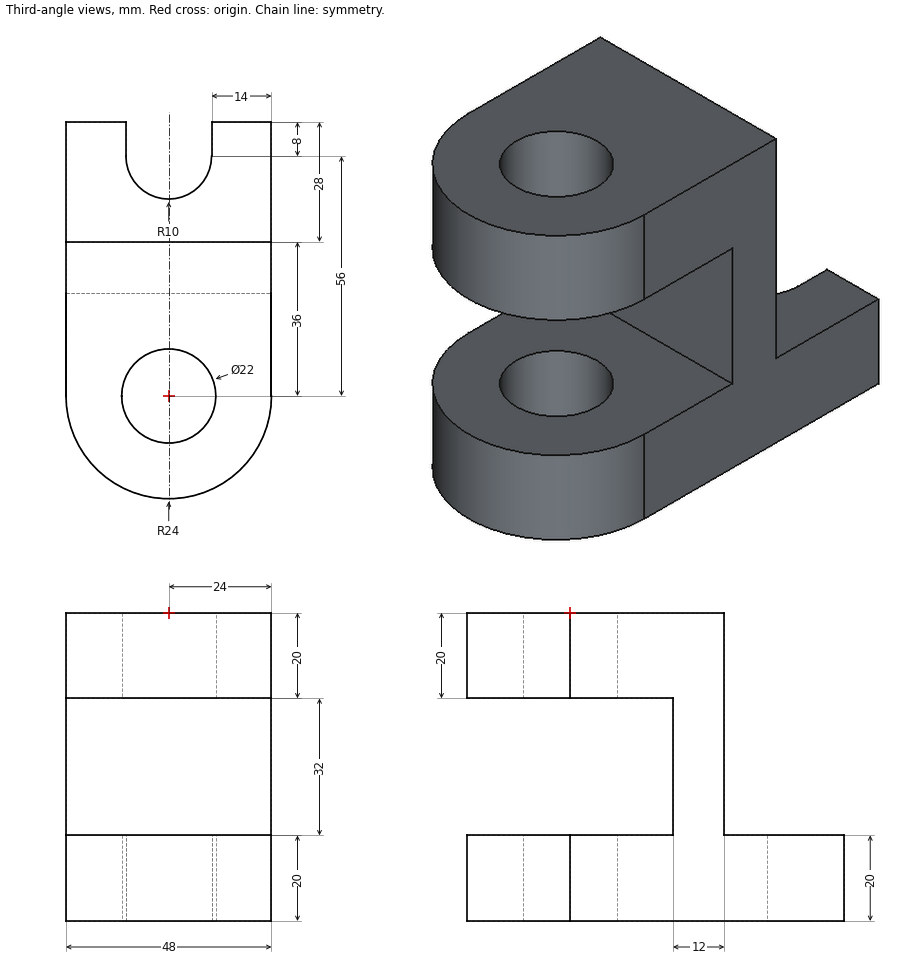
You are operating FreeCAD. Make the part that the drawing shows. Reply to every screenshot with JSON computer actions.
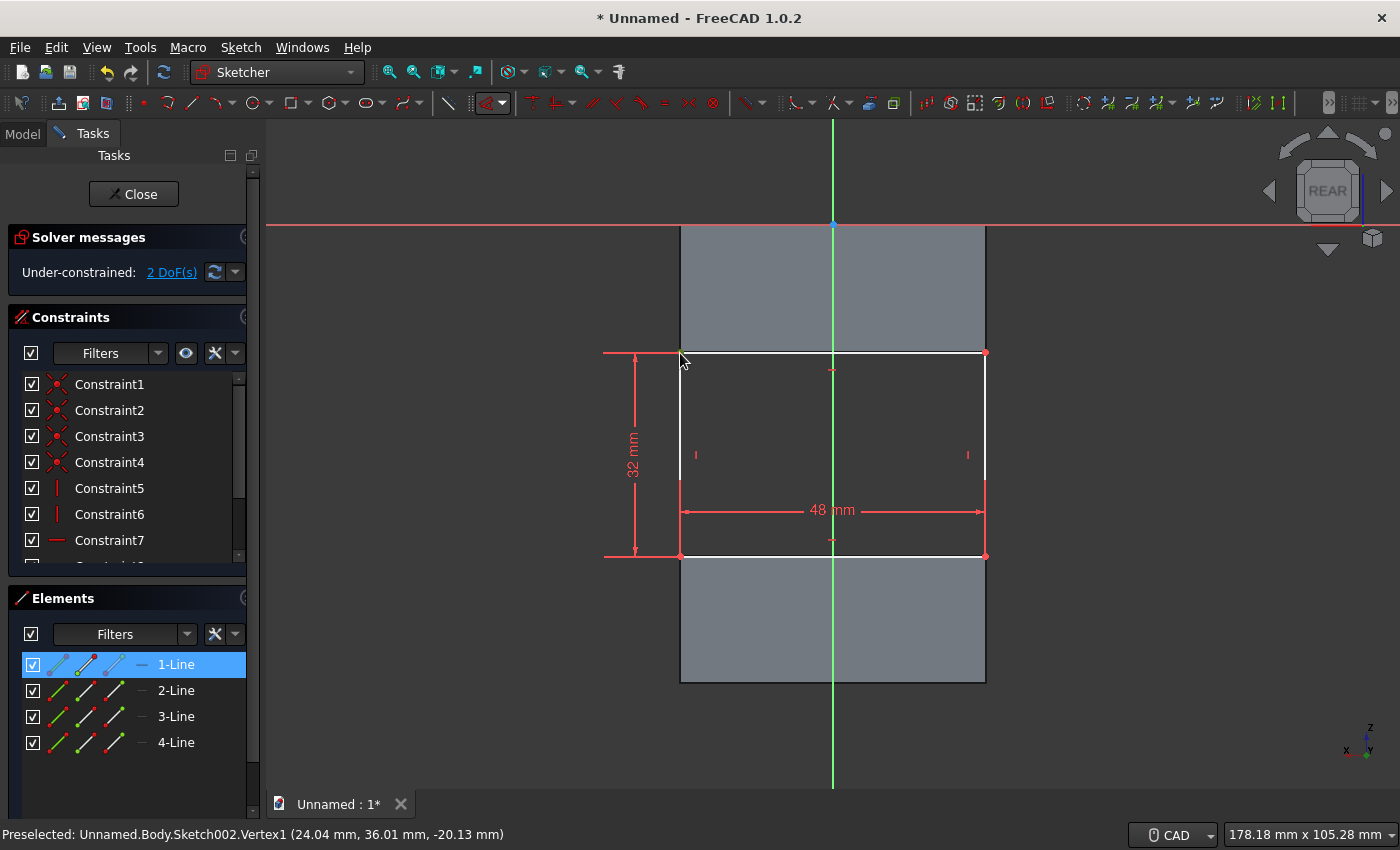
{"action": "left_click", "coordinate": [504, 104]}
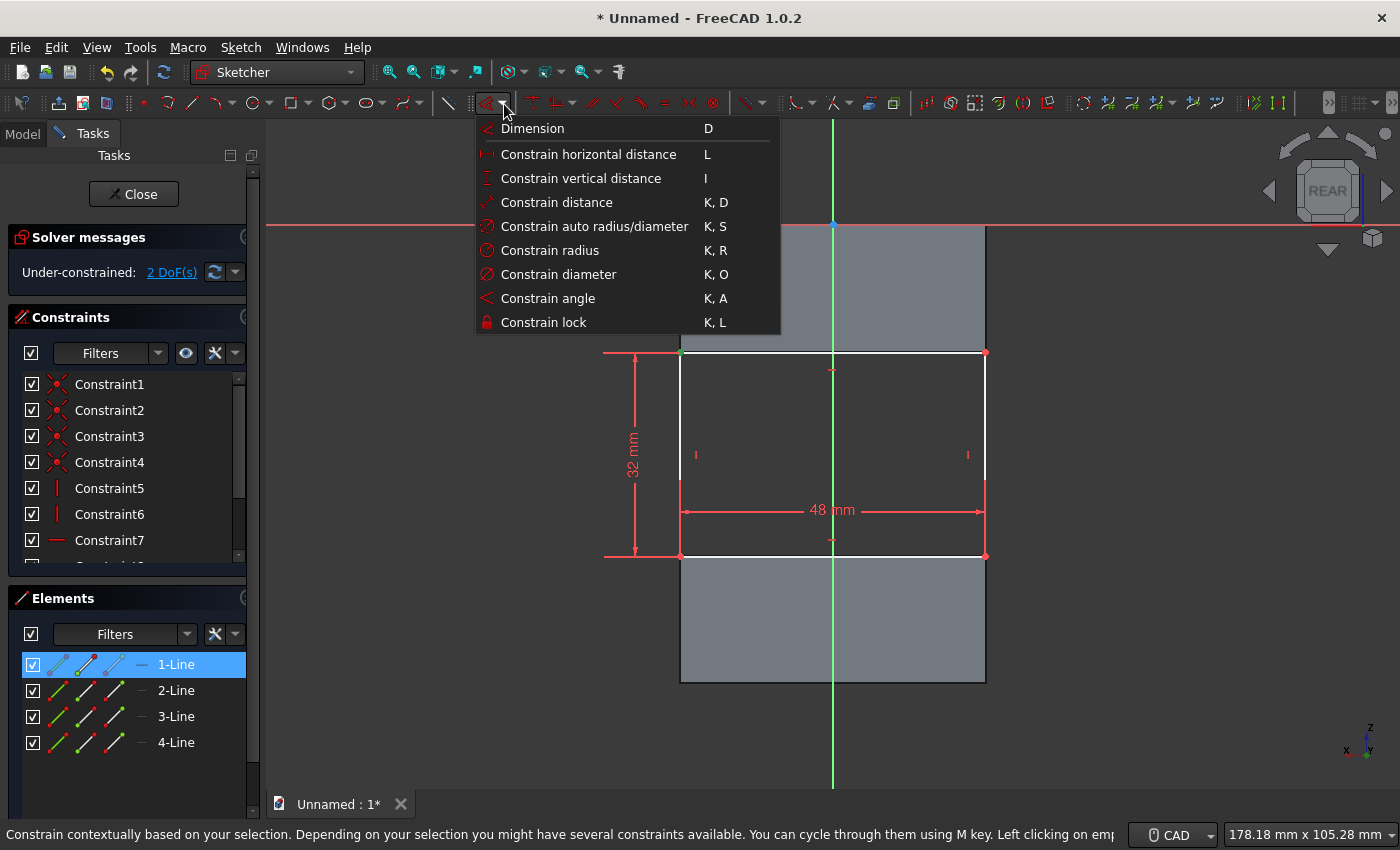
{"action": "left_click", "coordinate": [628, 154]}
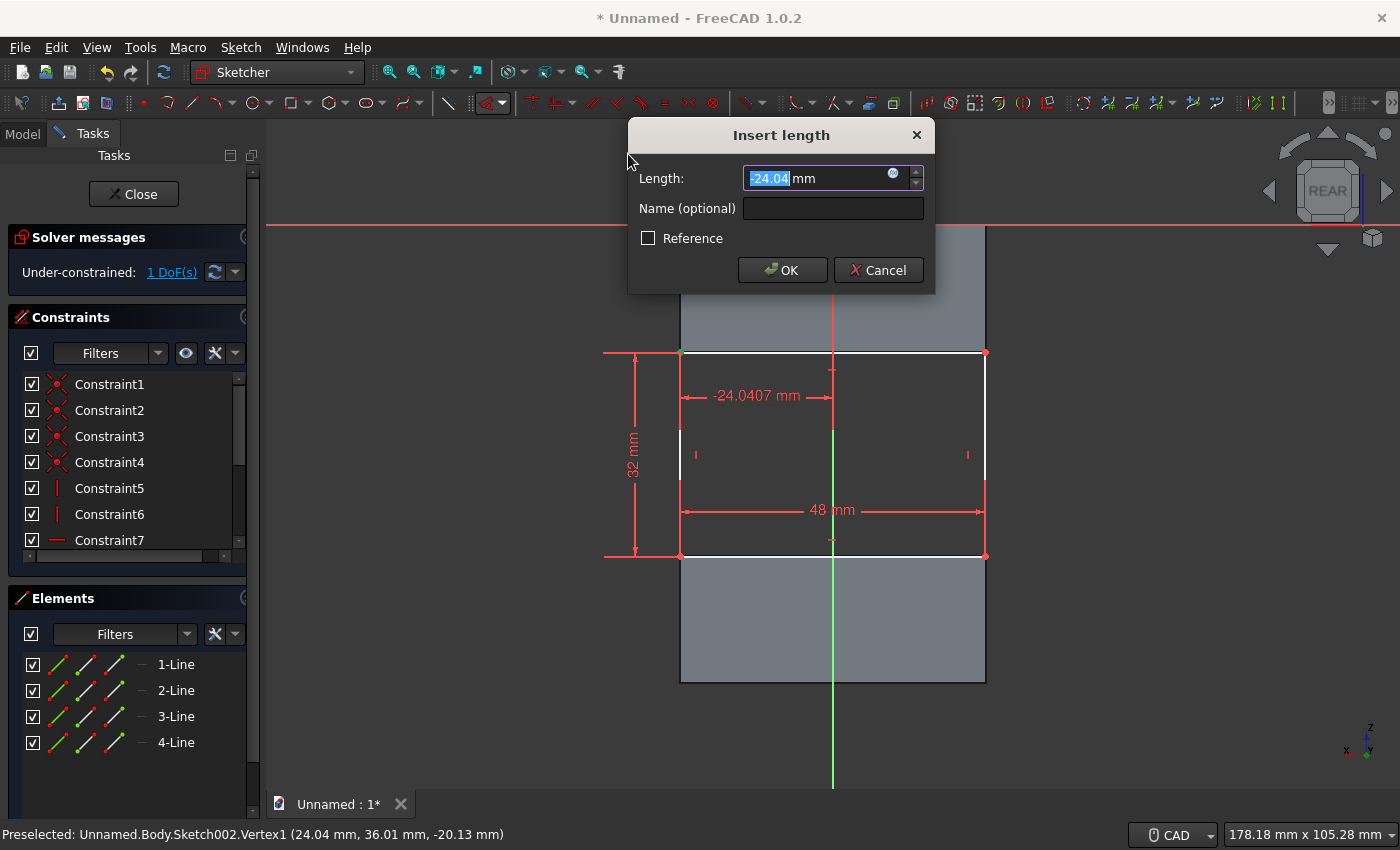
{"action": "type", "text": "-24"}
{"action": "key", "text": "Return"}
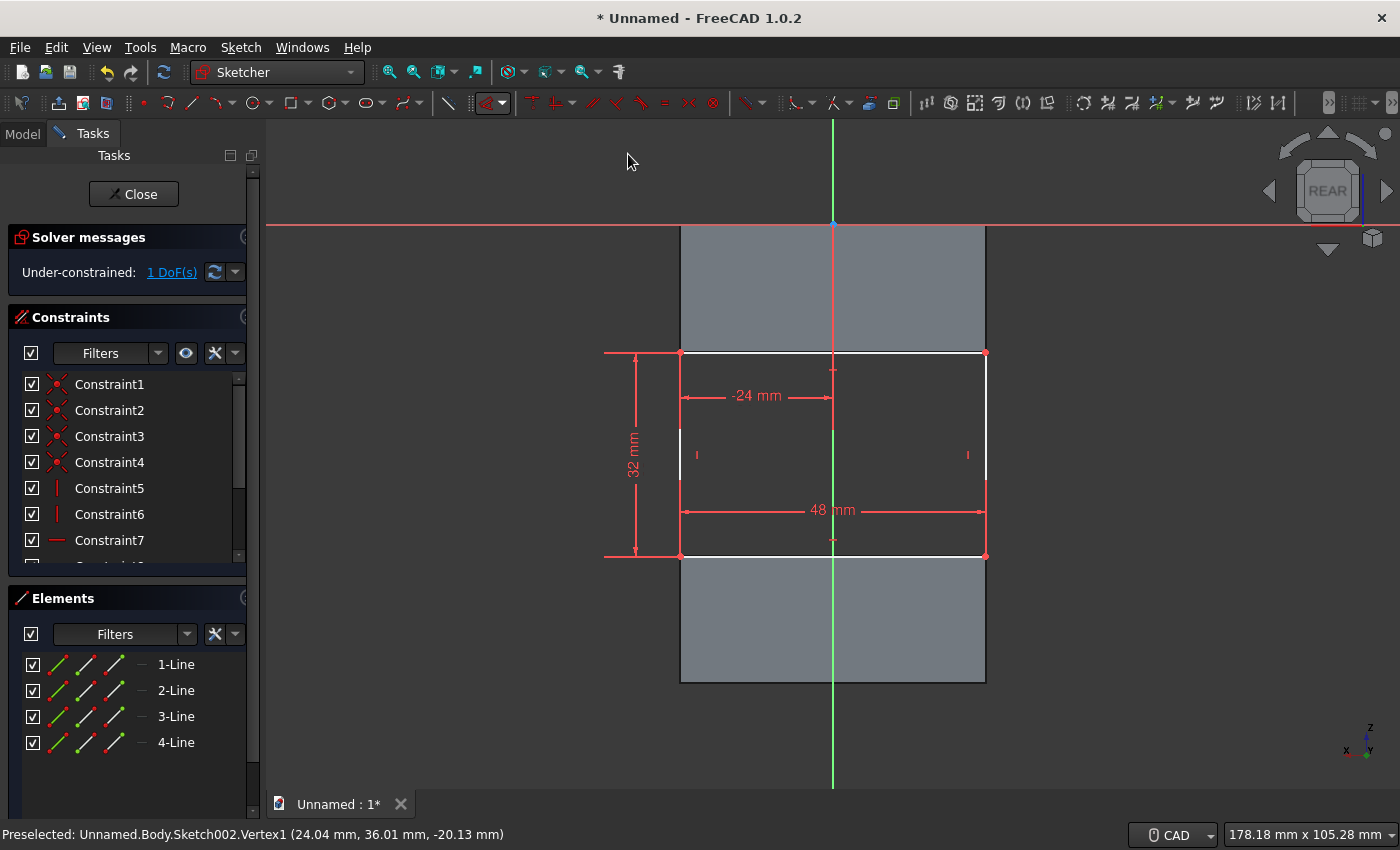
{"action": "left_click", "coordinate": [680, 353]}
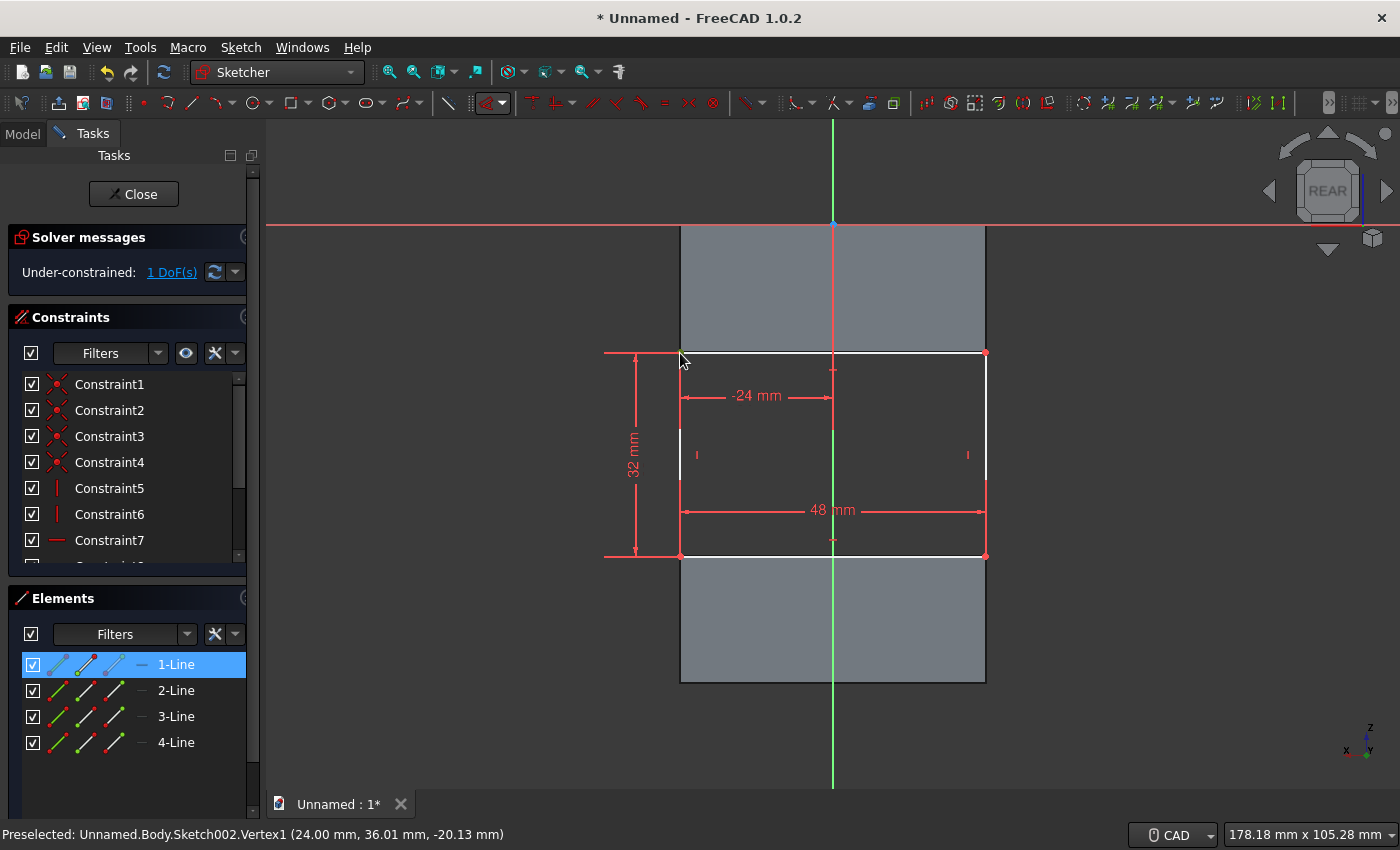
{"action": "left_click", "coordinate": [504, 104]}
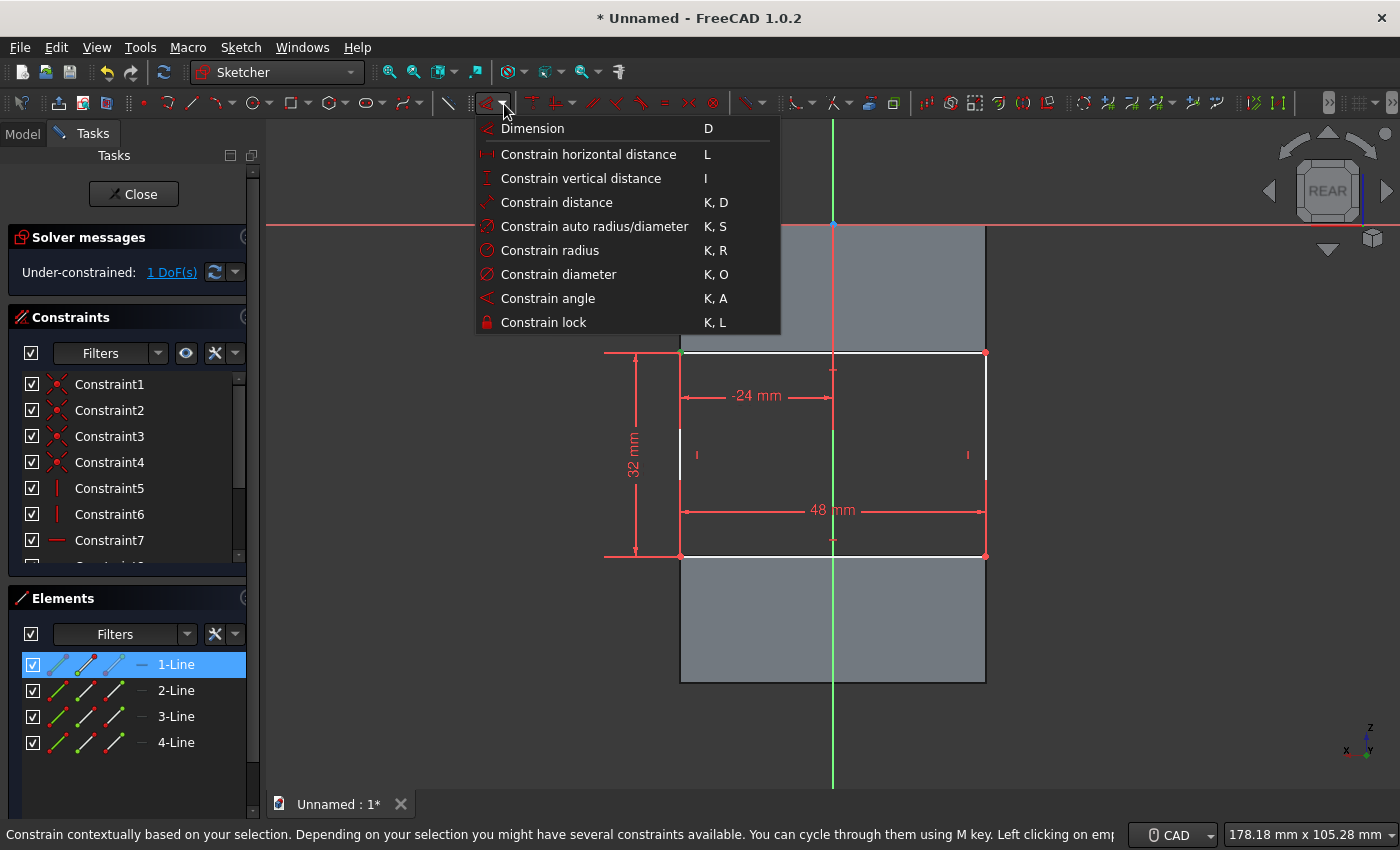
{"action": "left_click", "coordinate": [628, 178]}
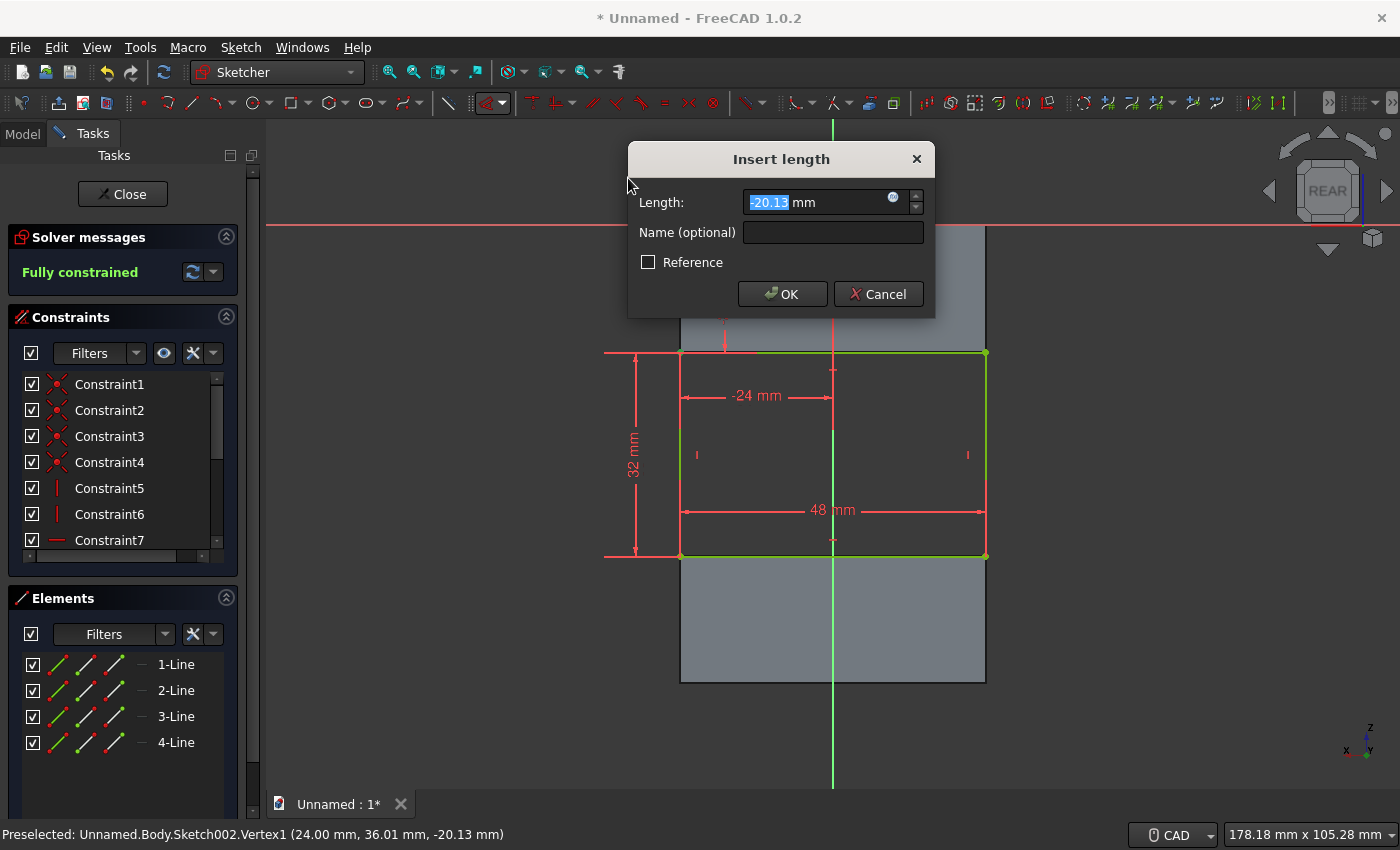
{"action": "type", "text": "-20"}
{"action": "key", "text": "Return"}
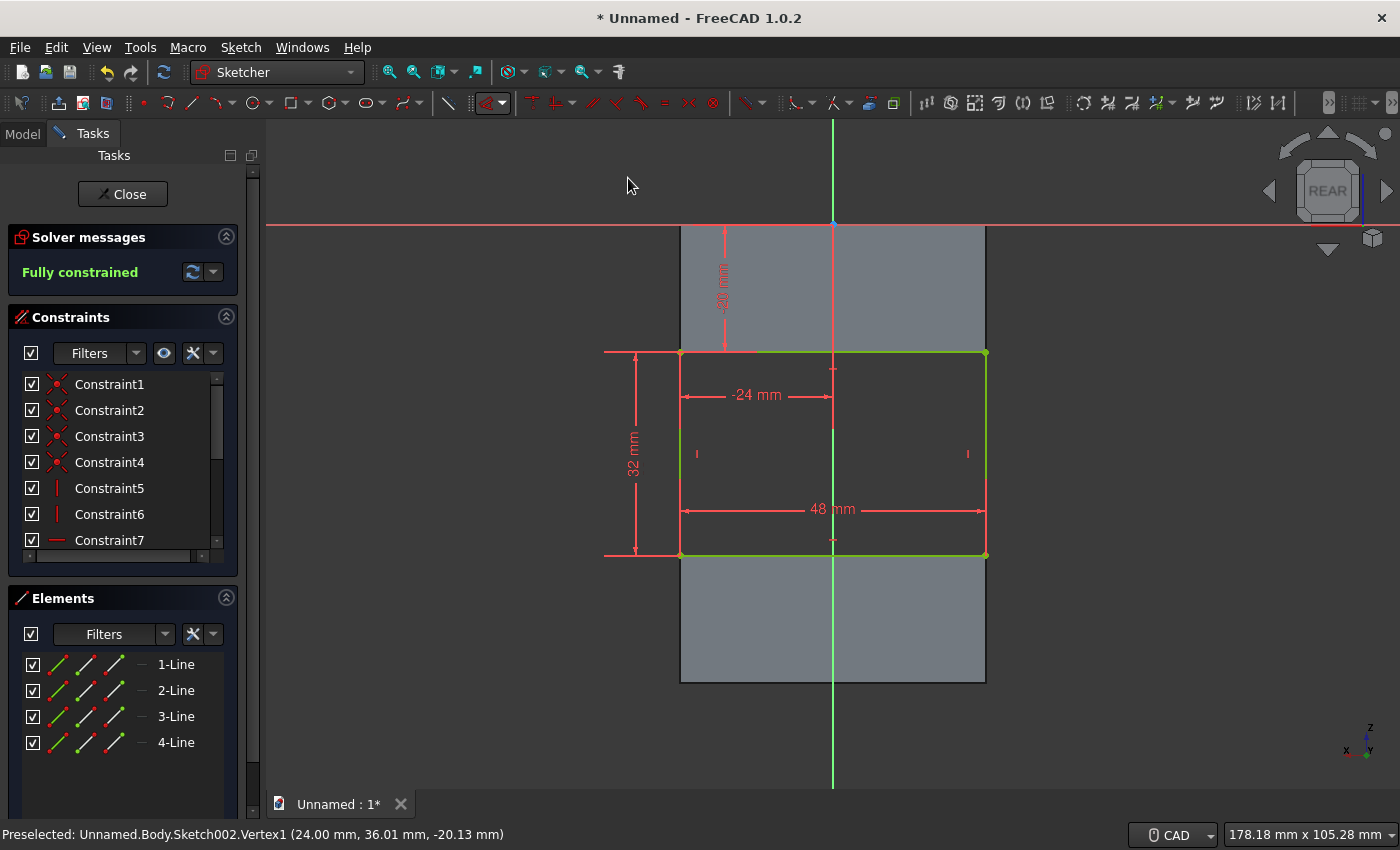
{"action": "left_click", "coordinate": [123, 194]}